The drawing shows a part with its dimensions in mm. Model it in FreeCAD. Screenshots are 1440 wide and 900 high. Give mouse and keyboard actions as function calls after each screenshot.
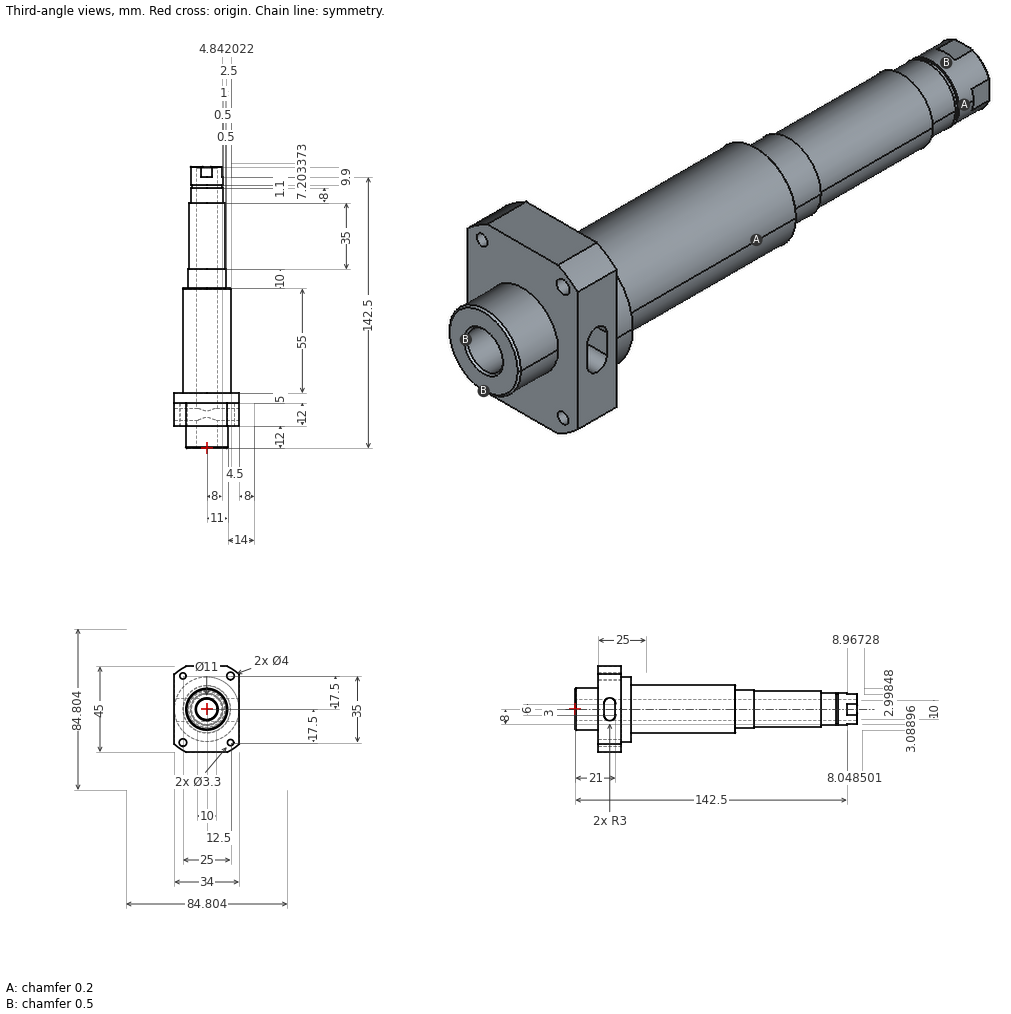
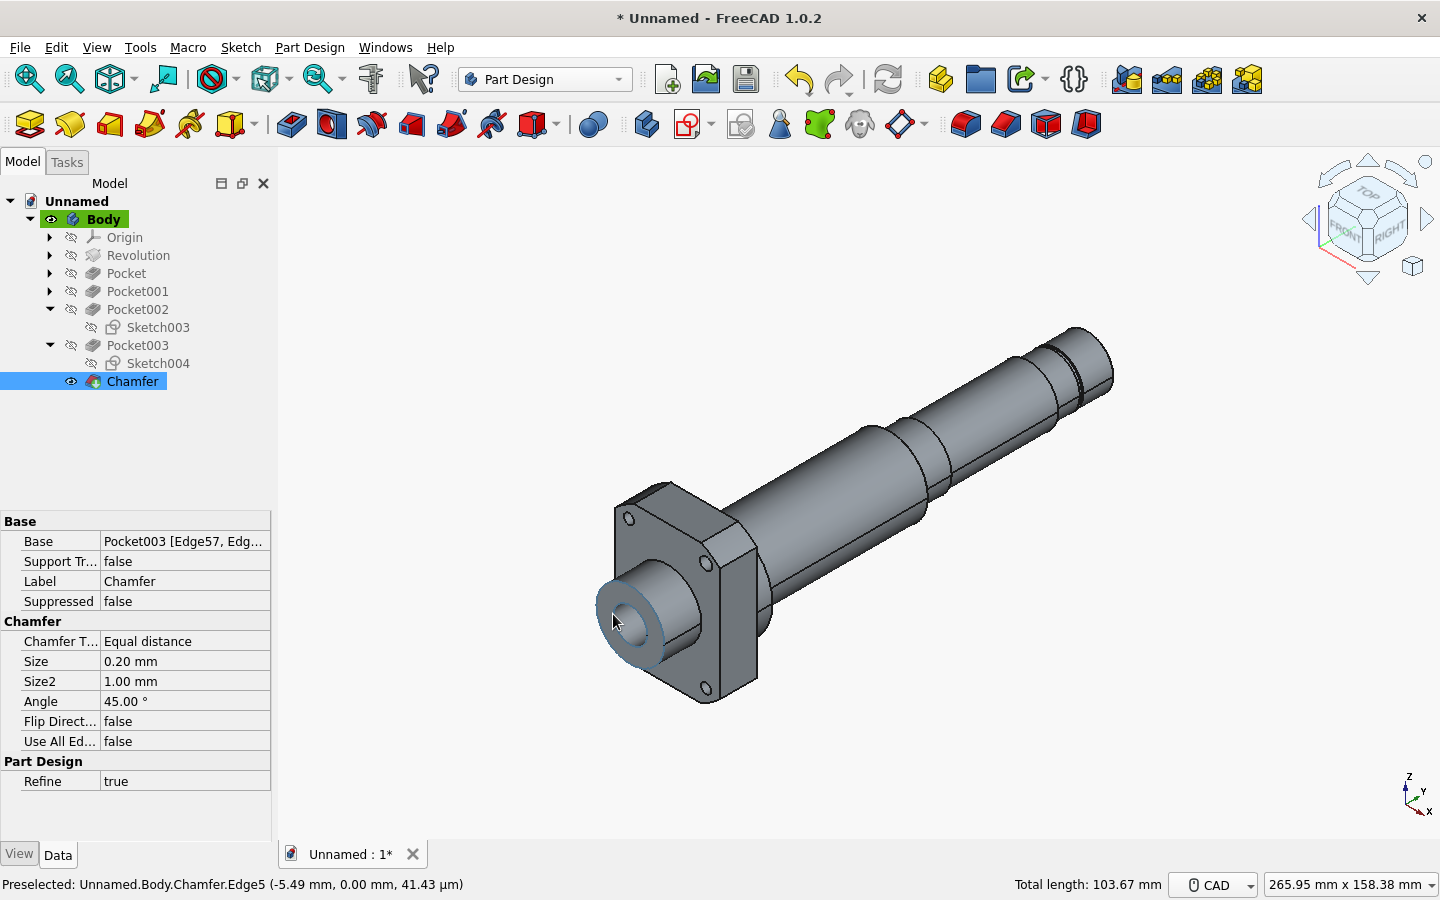
key(2)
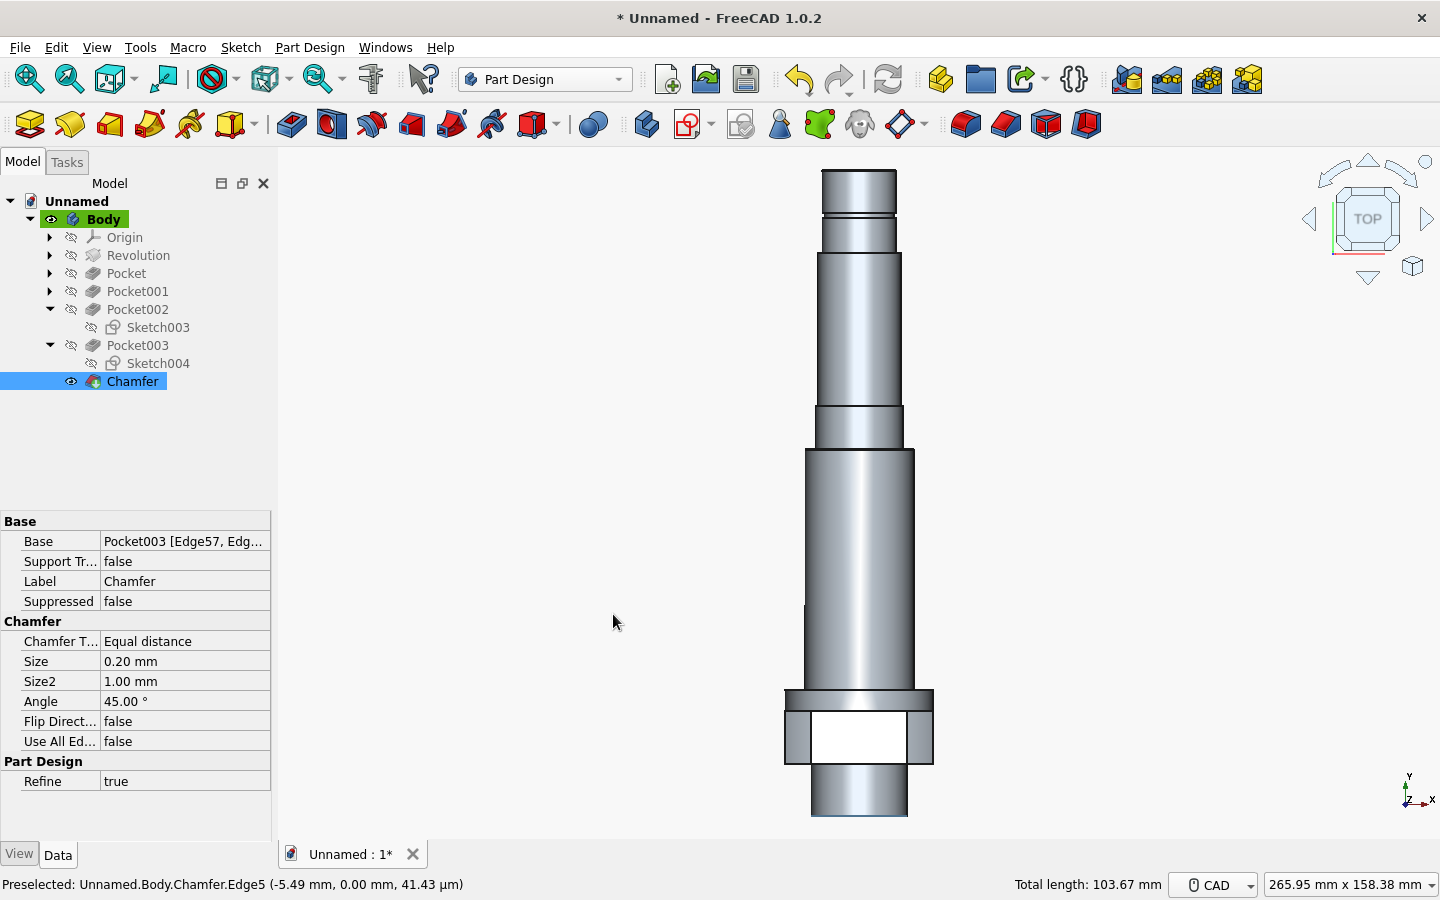
key(1)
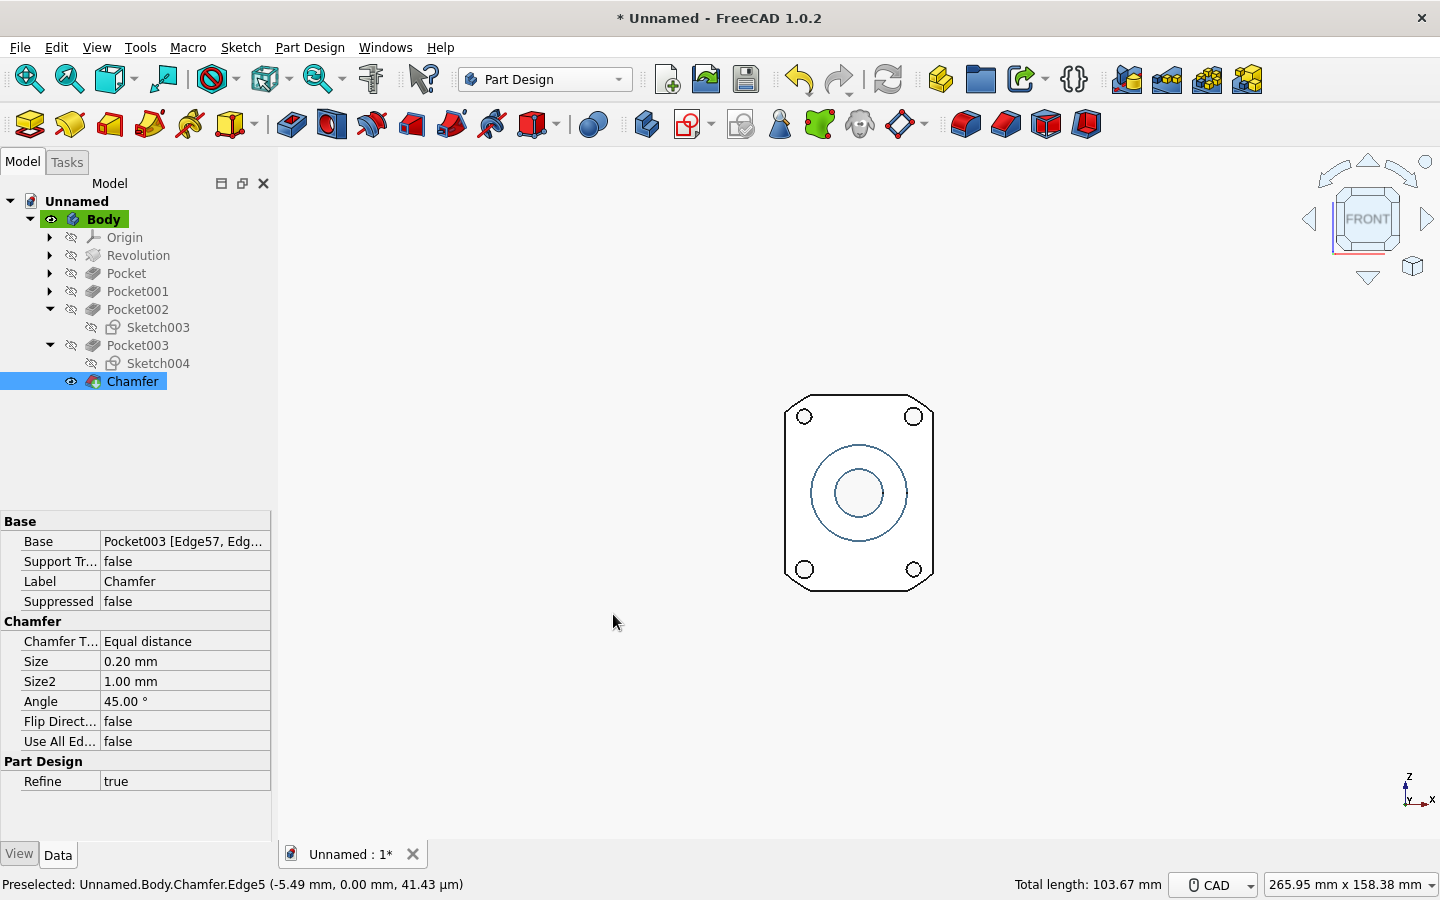
click(30, 80)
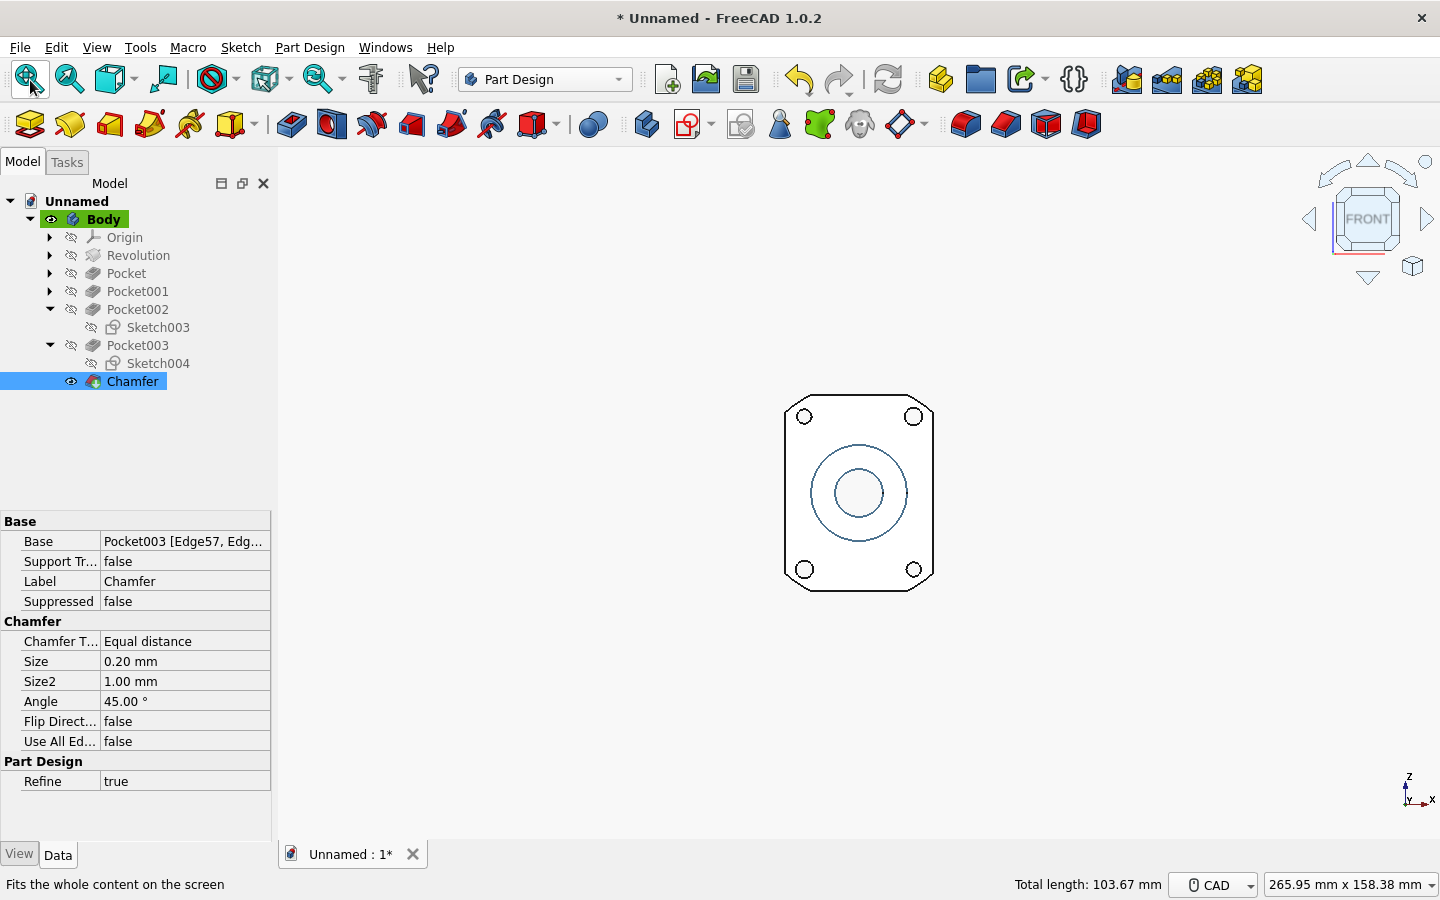
key(3)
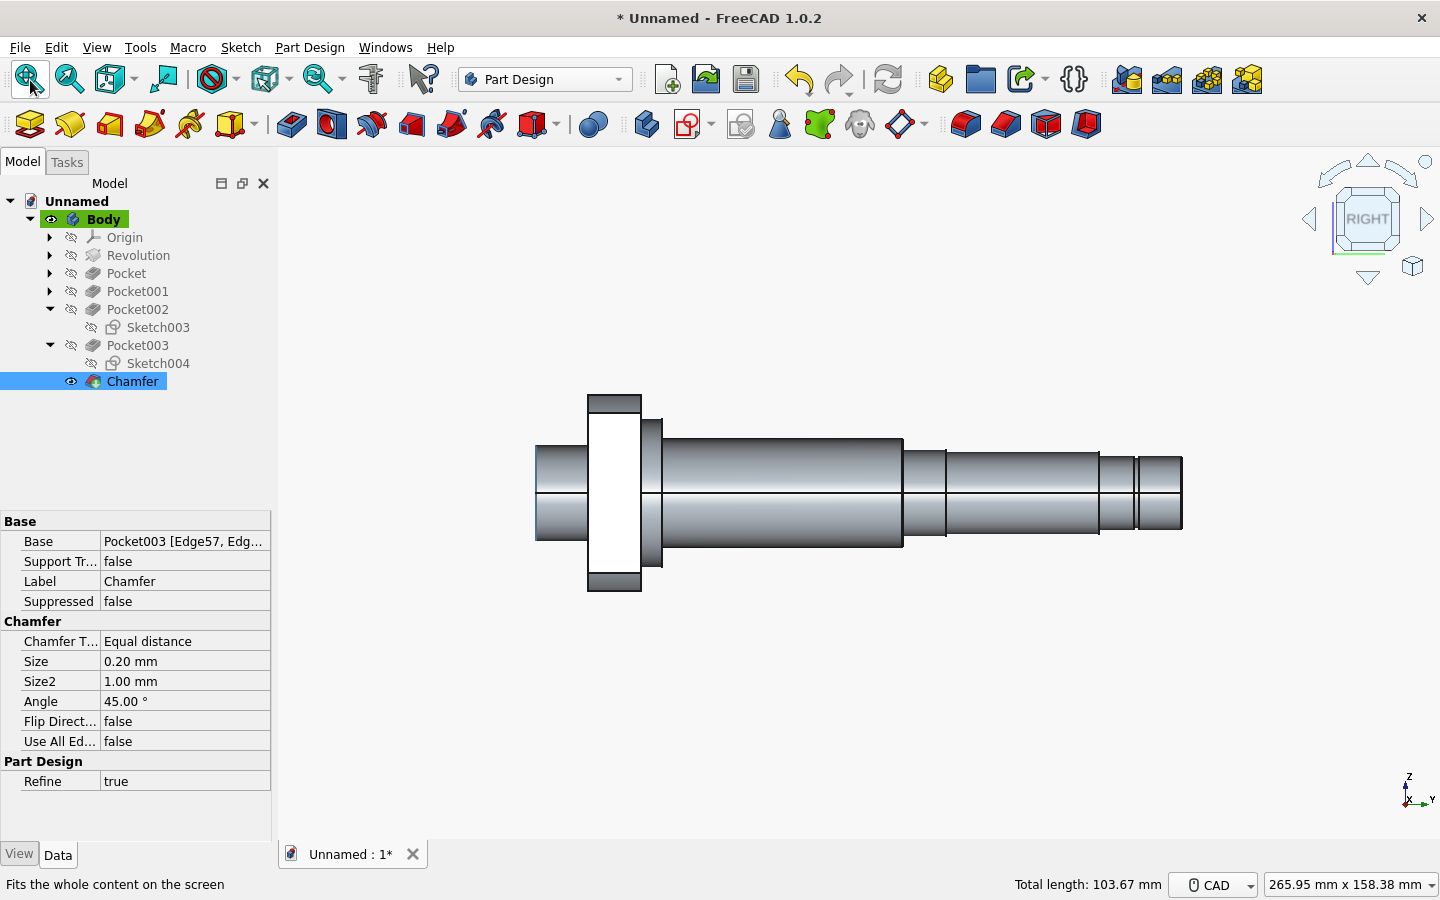
key(5)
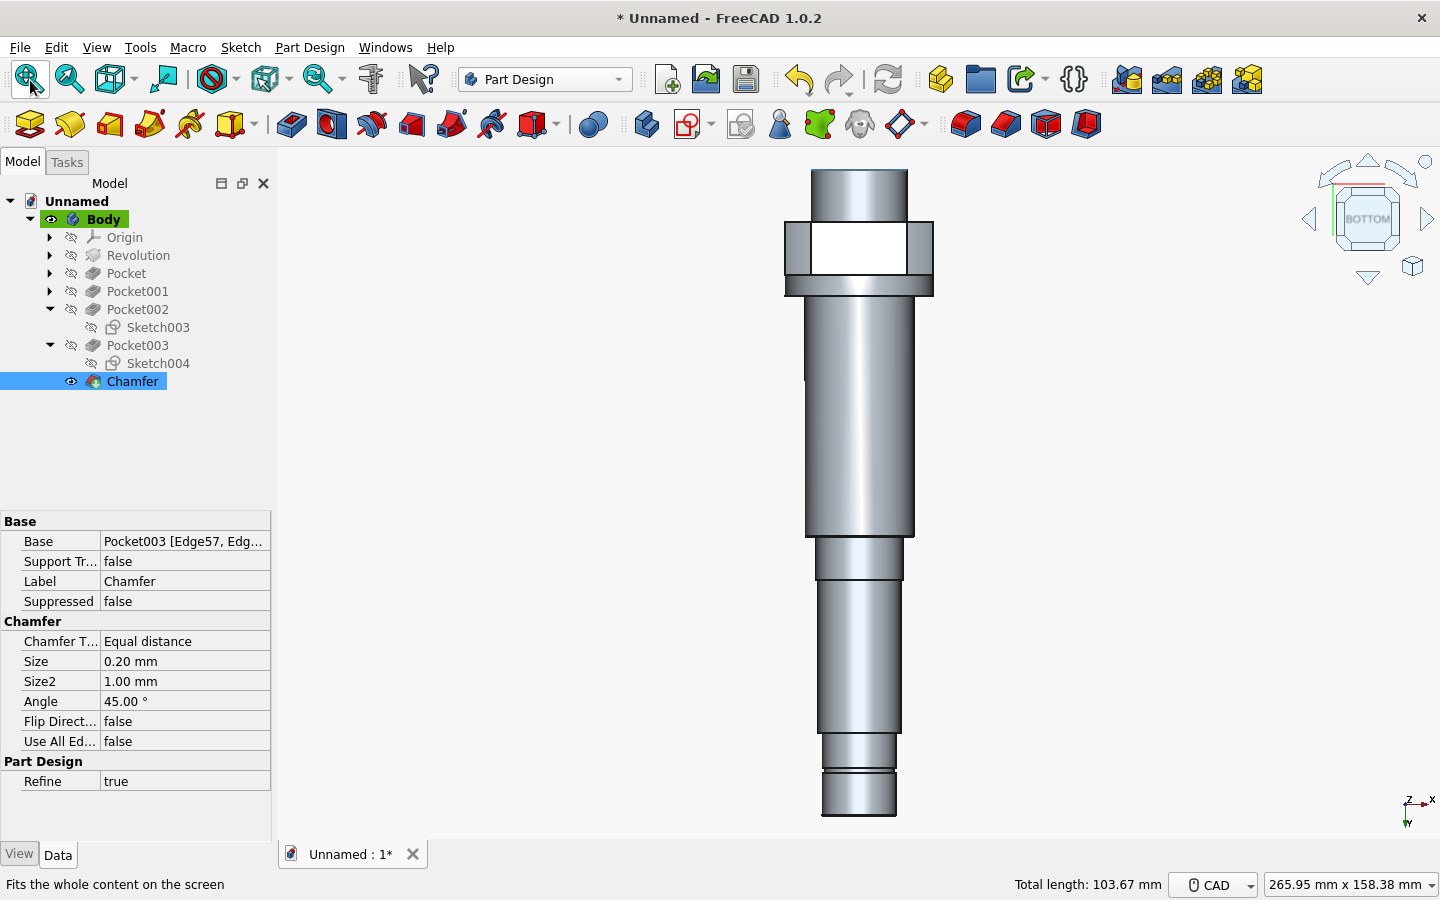
key(4)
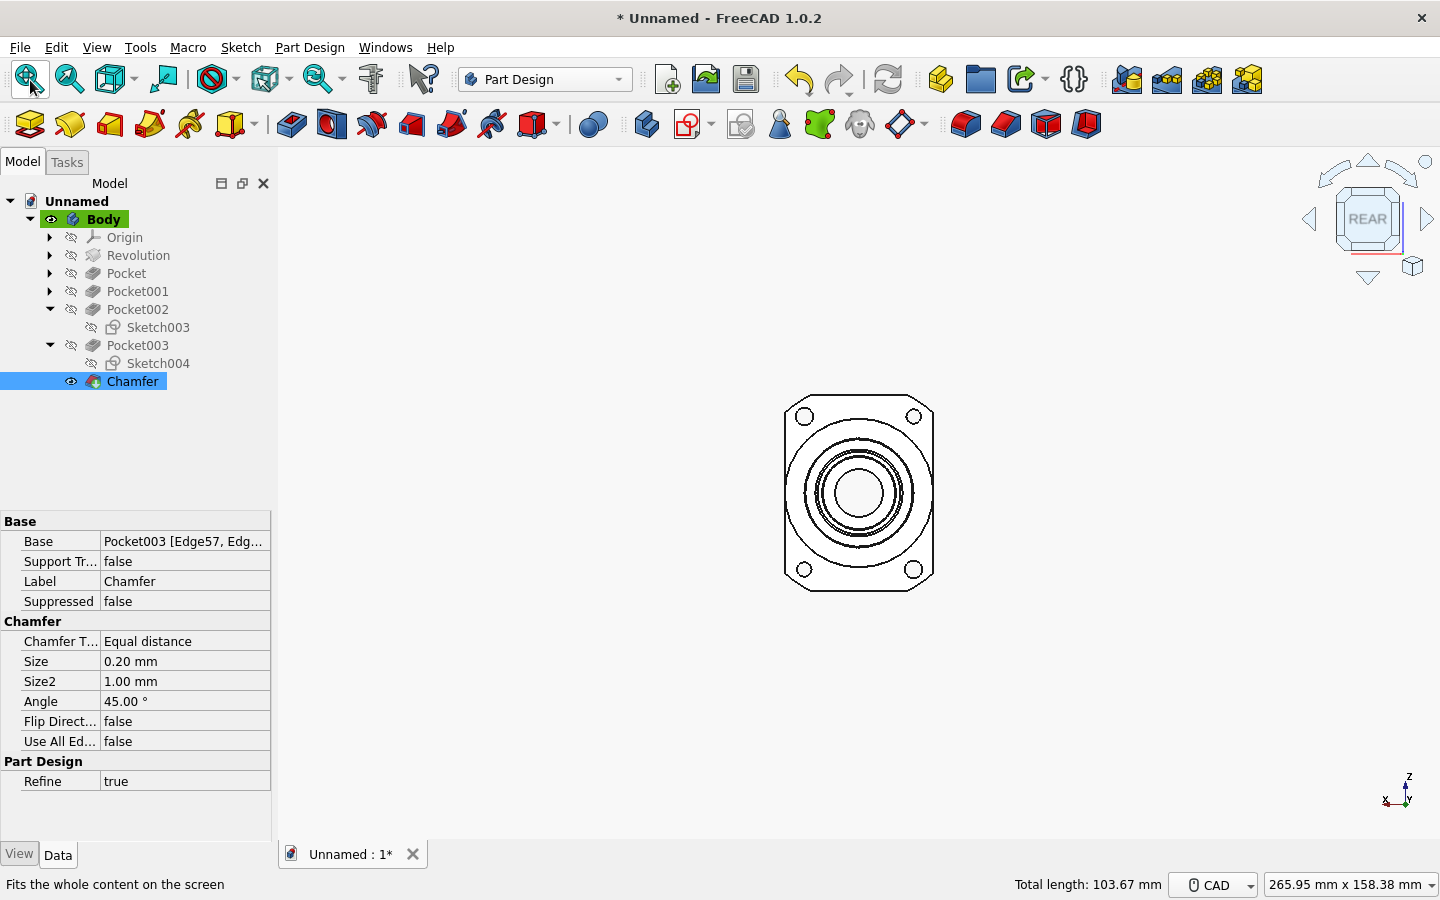
click(30, 80)